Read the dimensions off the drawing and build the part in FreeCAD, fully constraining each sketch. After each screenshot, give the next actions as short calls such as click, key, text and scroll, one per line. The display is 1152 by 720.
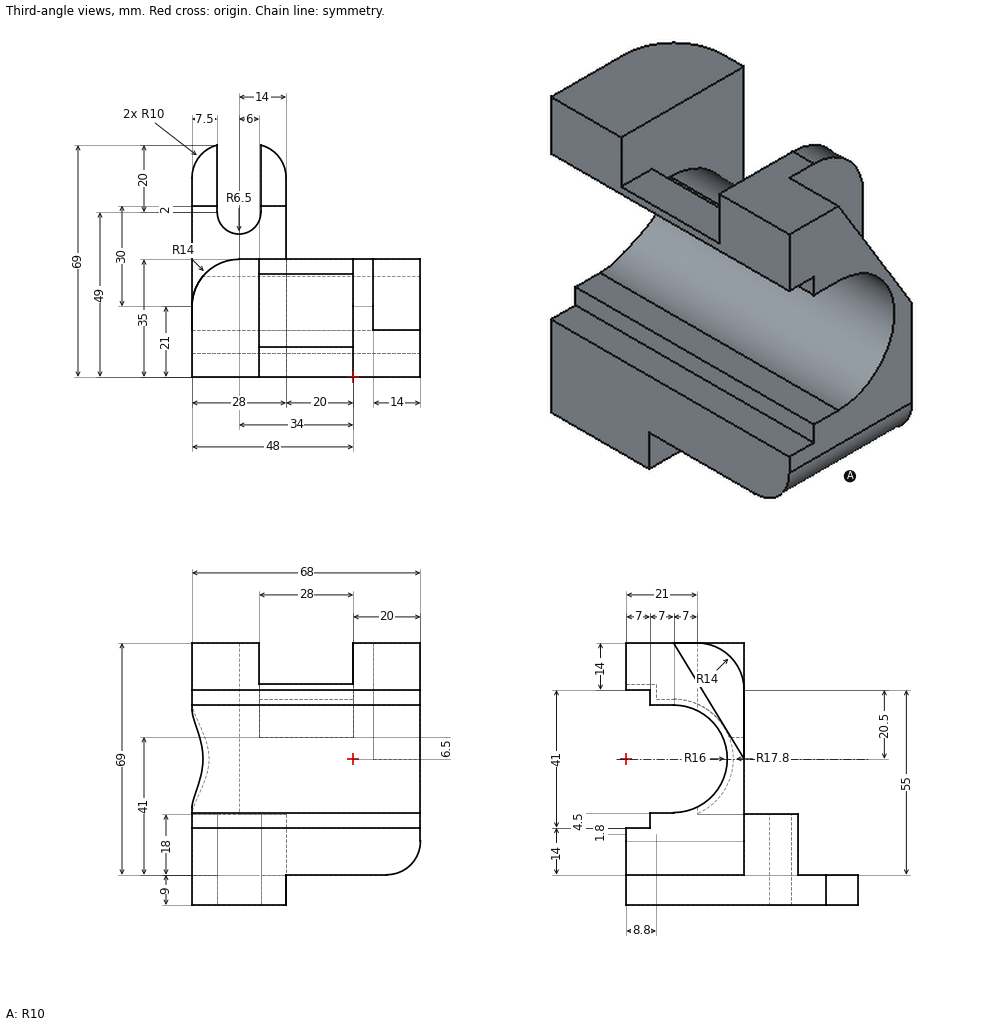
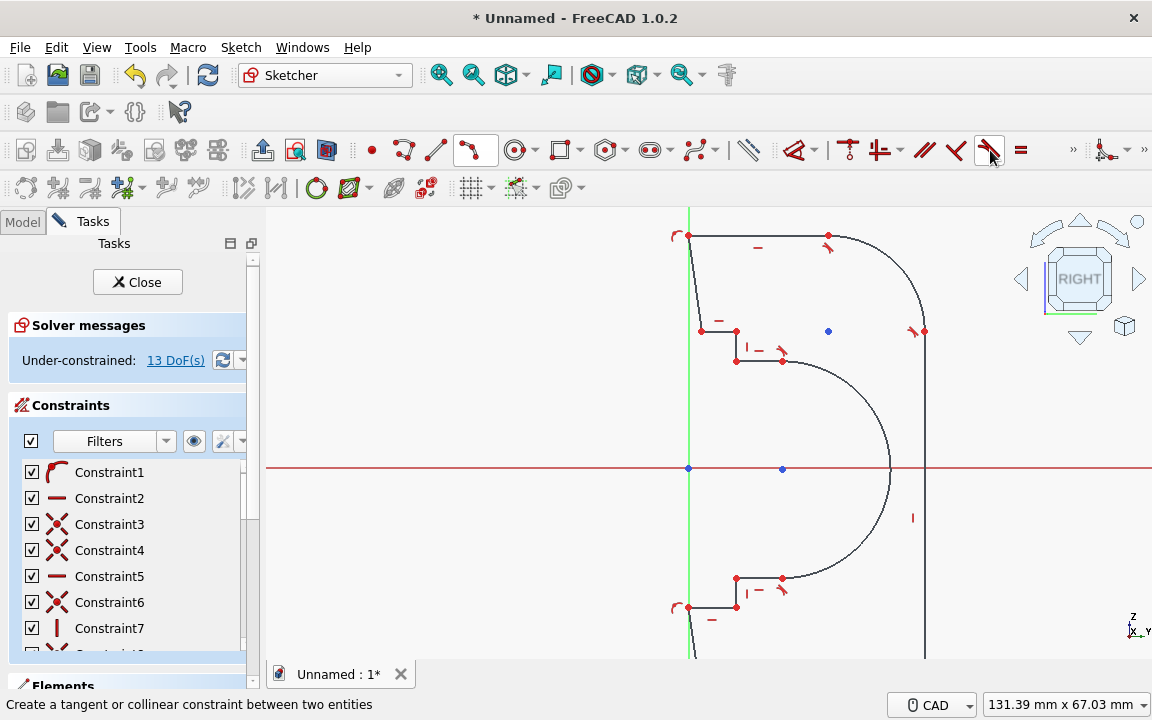
scroll(698, 303, up, 2)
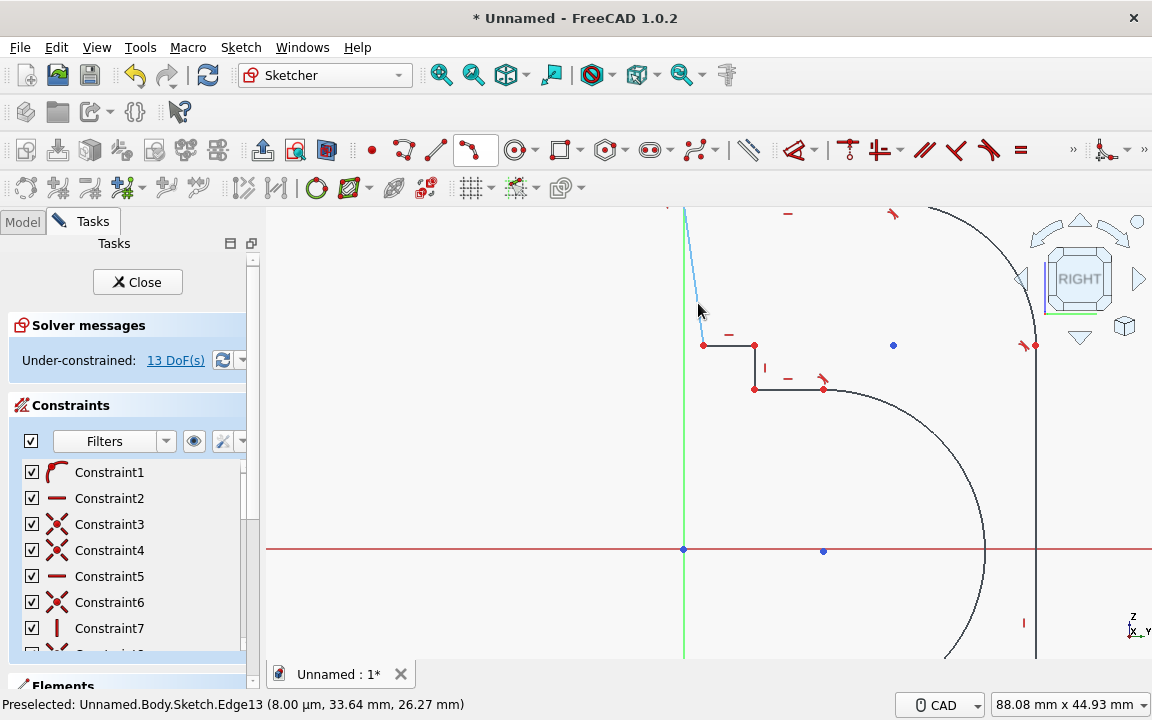
click(698, 303)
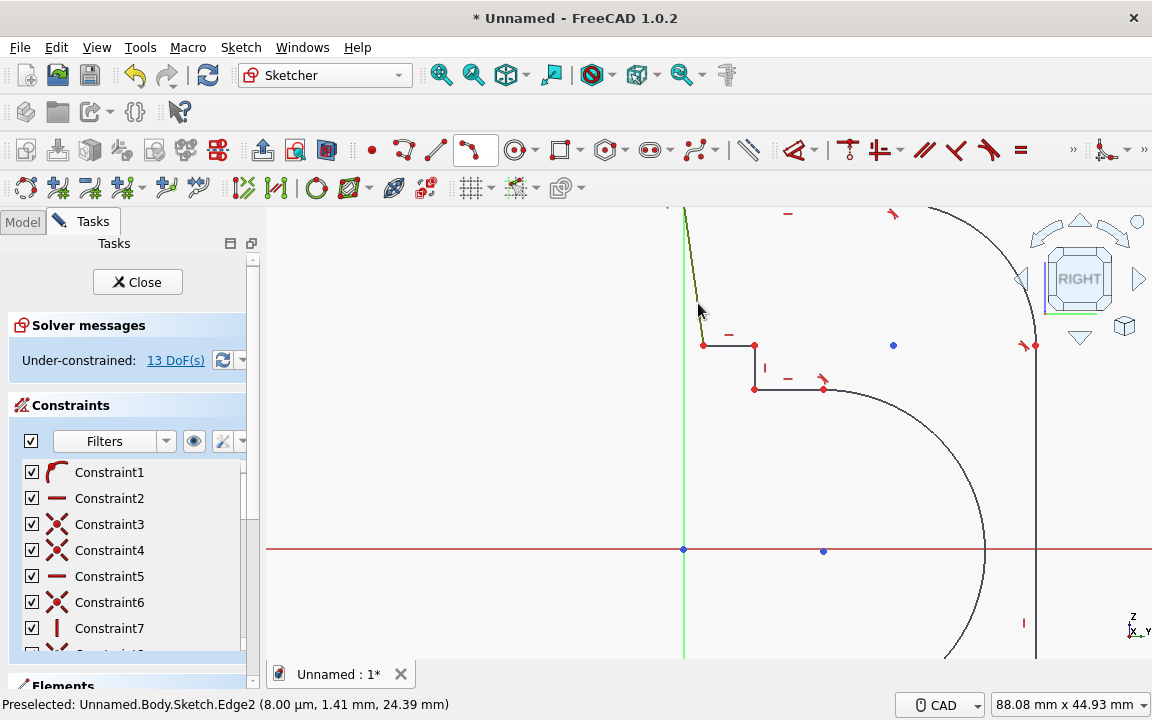
key(v)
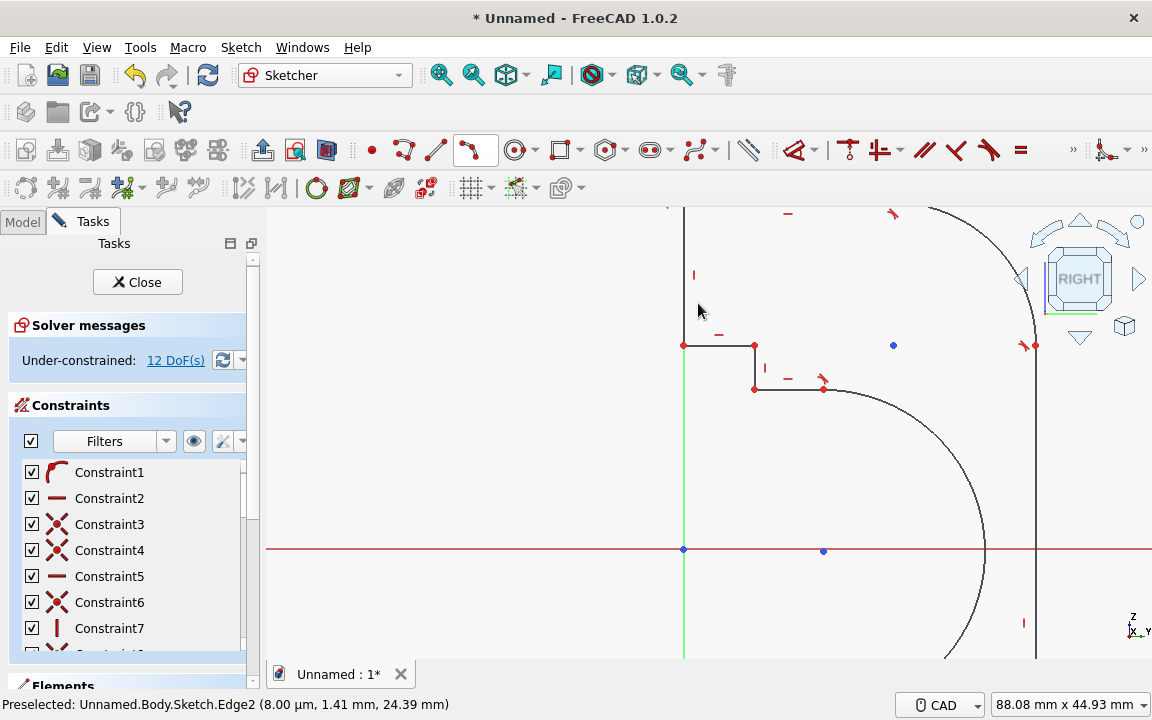
scroll(513, 365, down, 5)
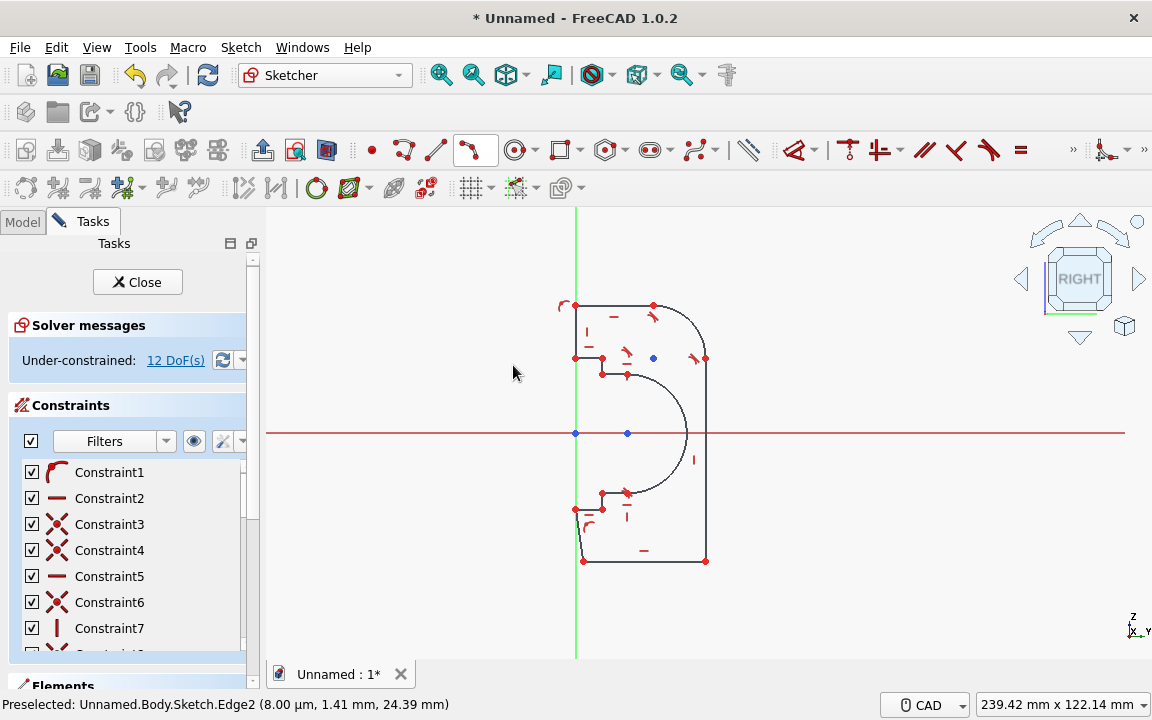
scroll(581, 546, up, 5)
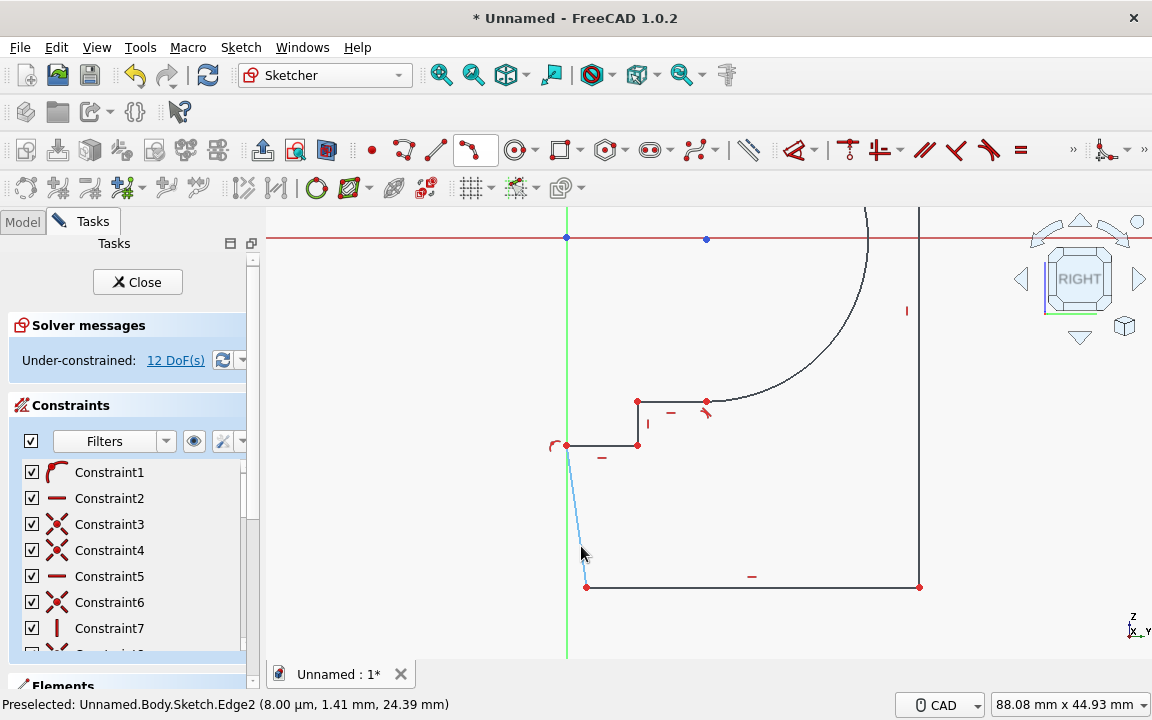
click(581, 545)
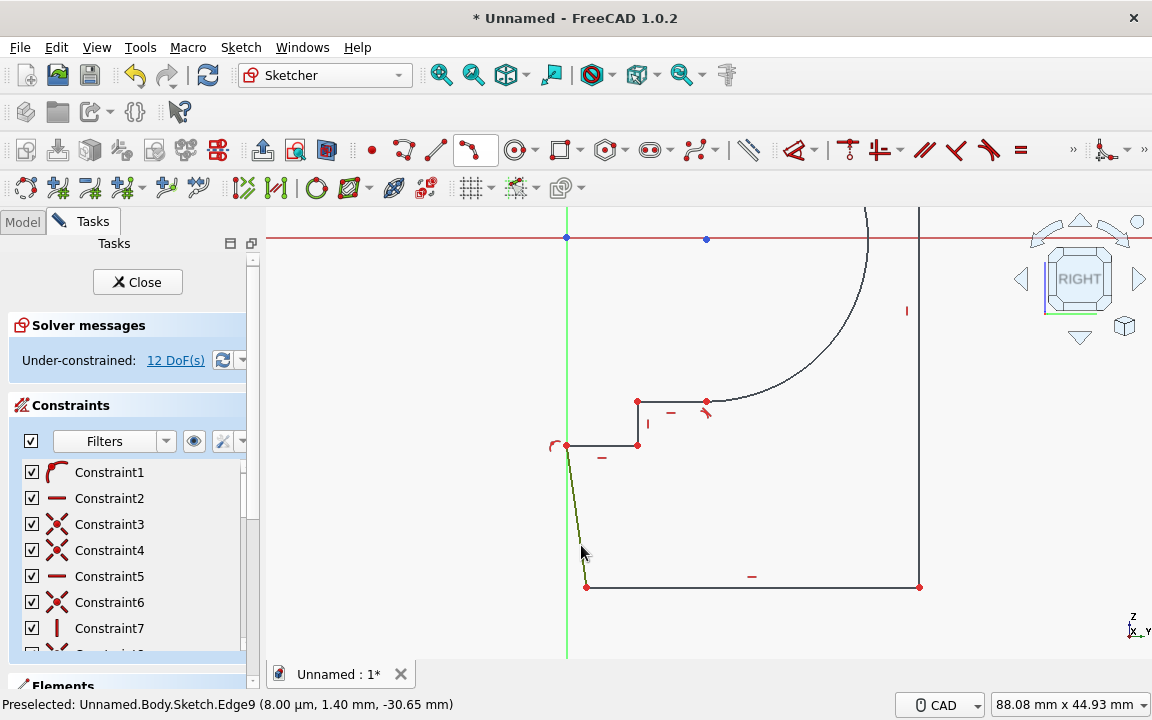
key(v)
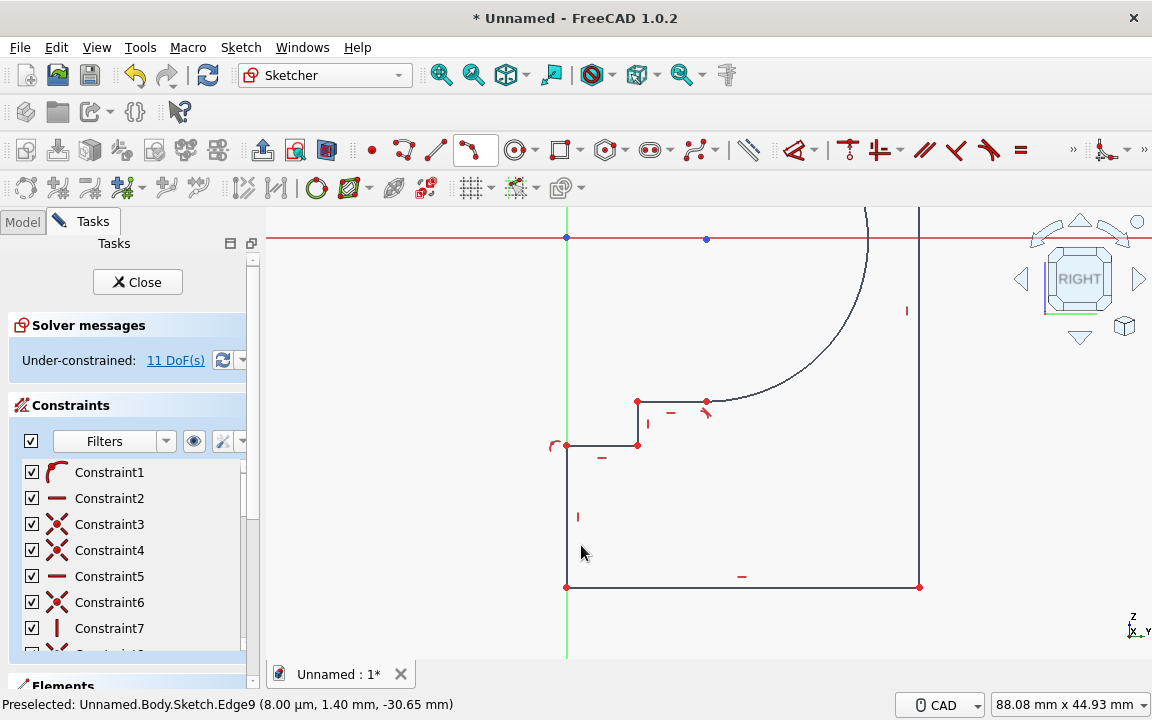
click(706, 240)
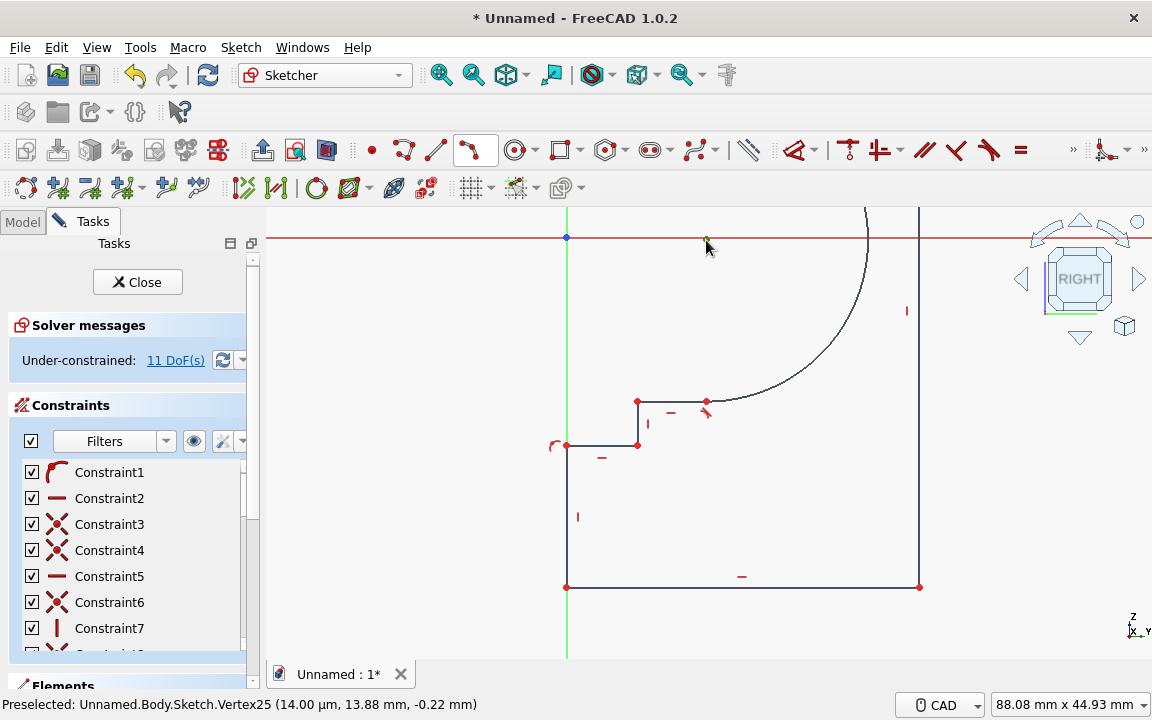
click(344, 238)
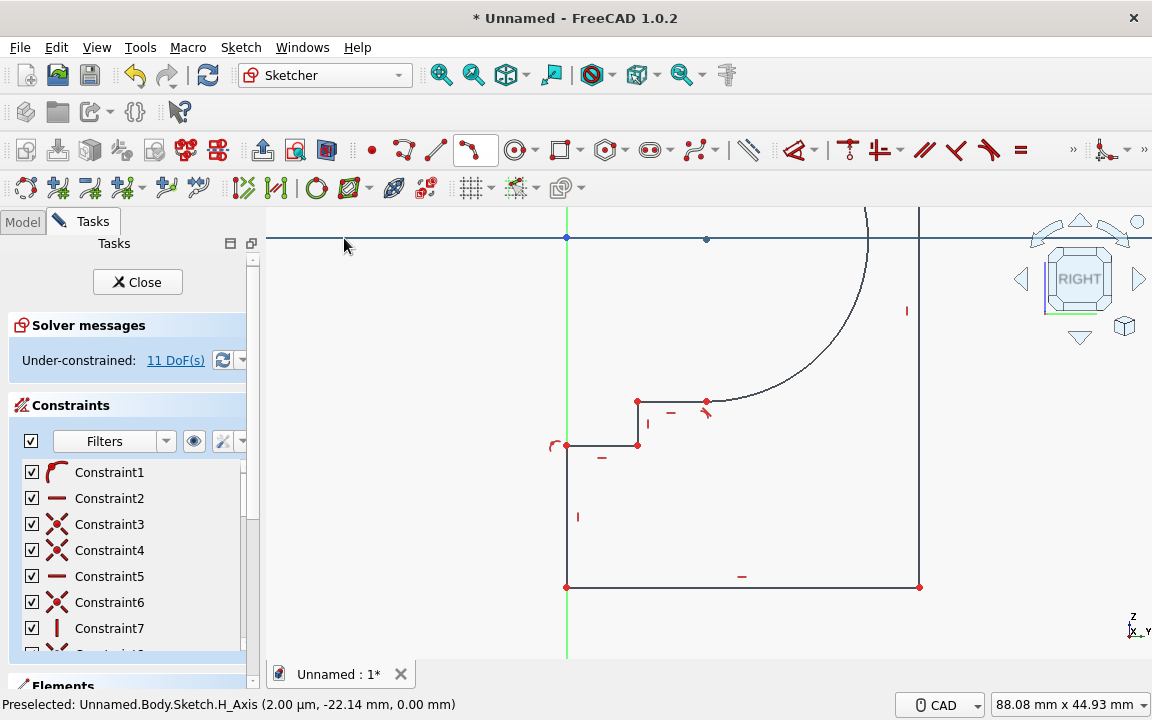
key(c)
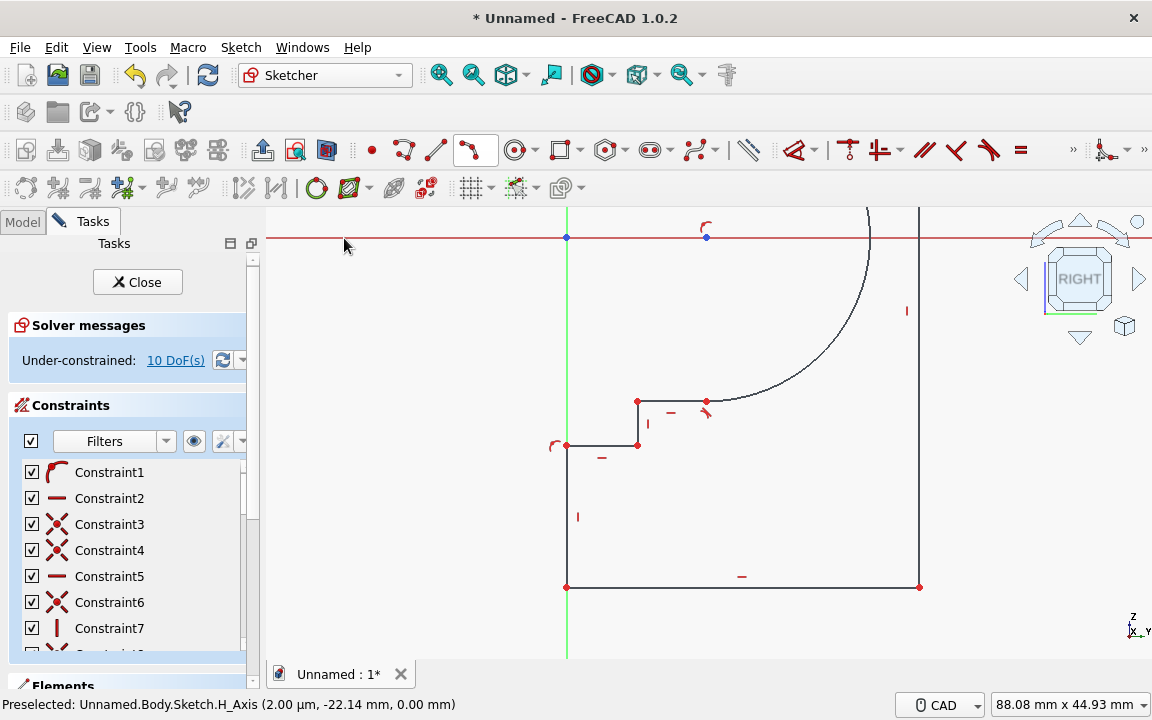
scroll(581, 547, down, 5)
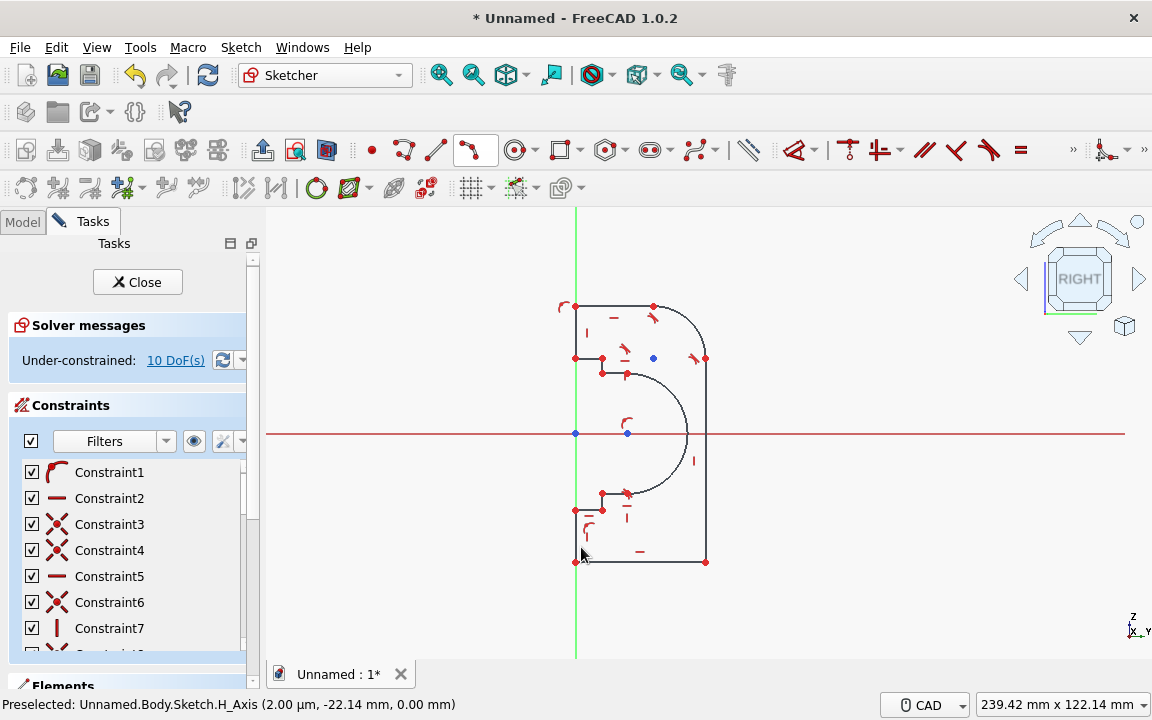
click(602, 359)